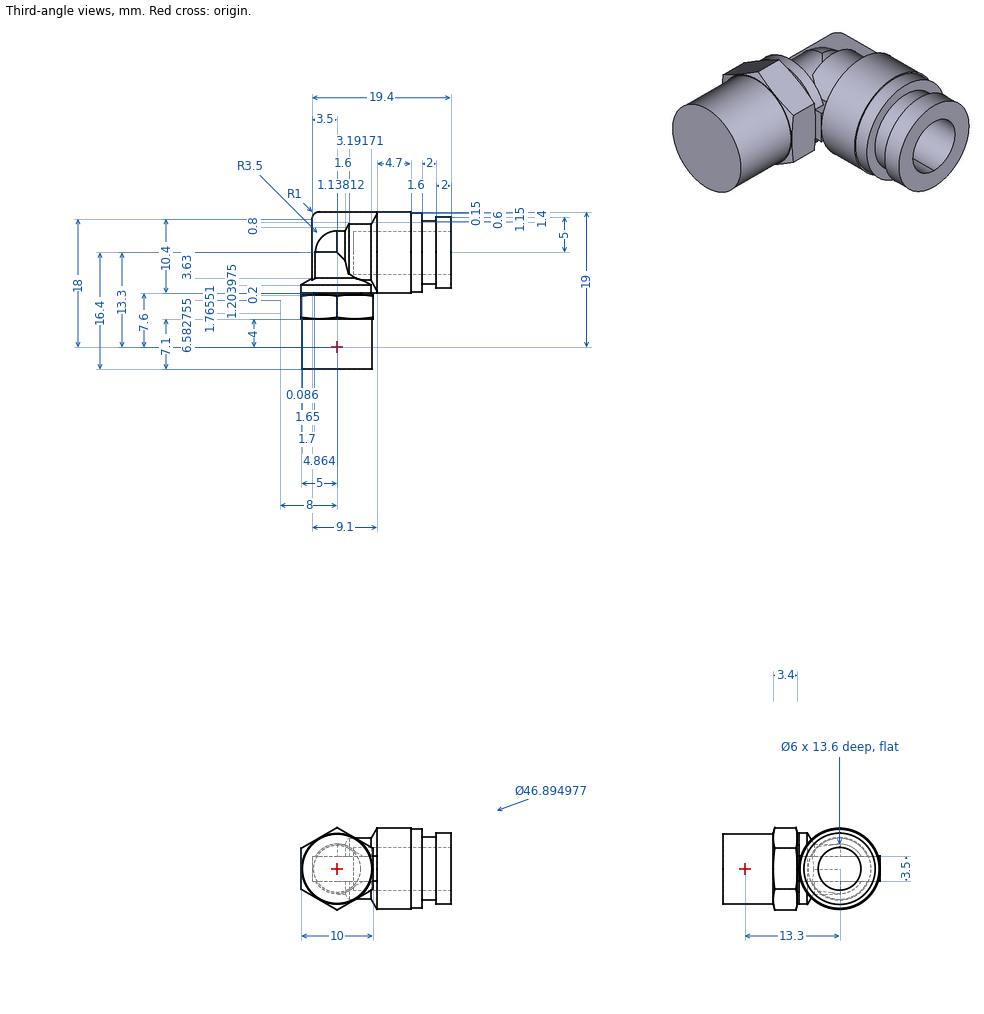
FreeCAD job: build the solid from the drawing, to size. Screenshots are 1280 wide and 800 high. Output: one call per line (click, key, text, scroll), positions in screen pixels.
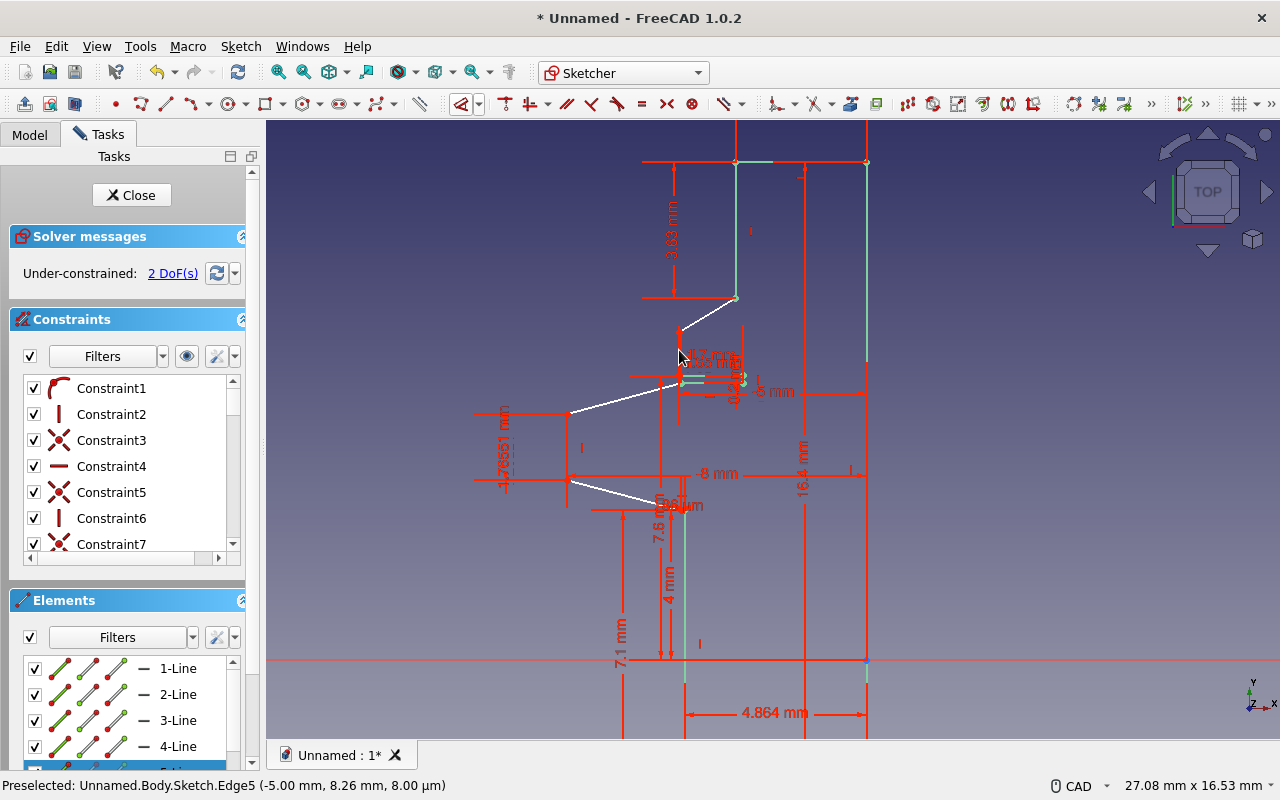
key(i)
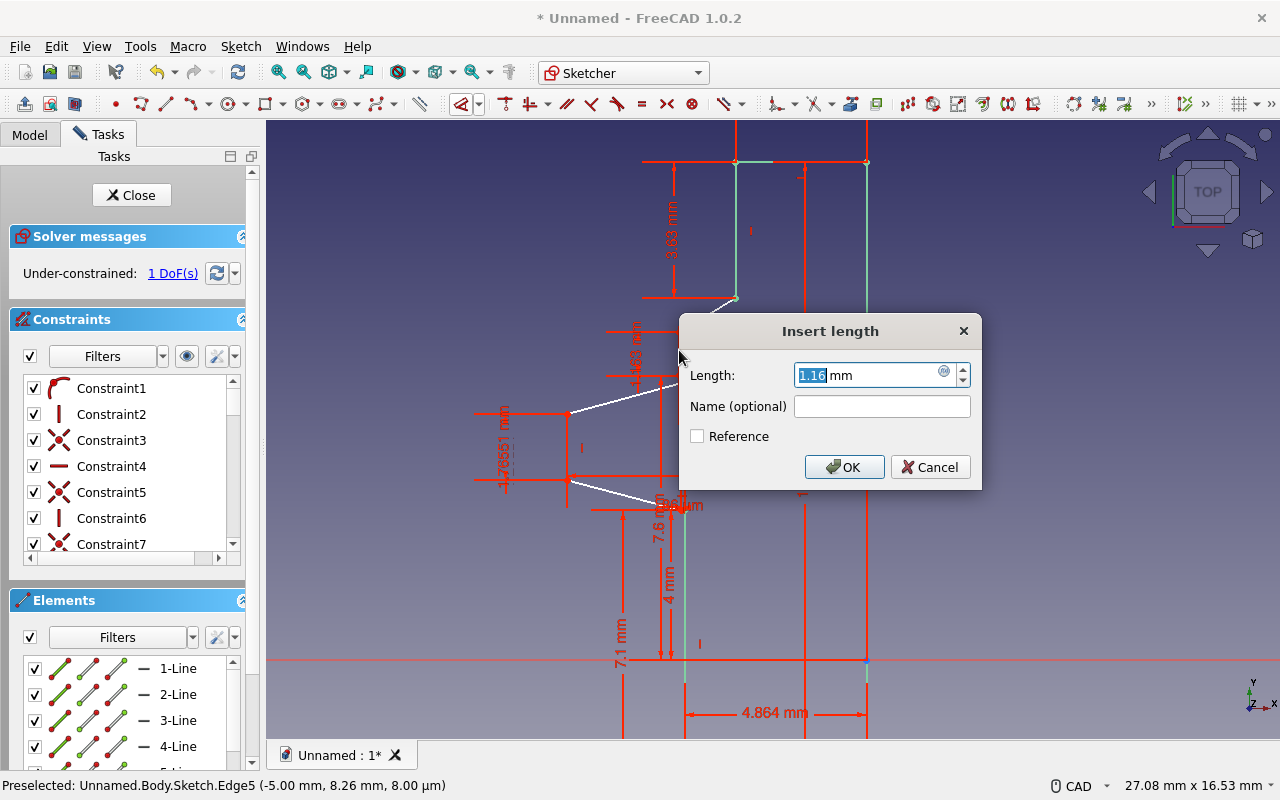
text(1.203975)
key(Return)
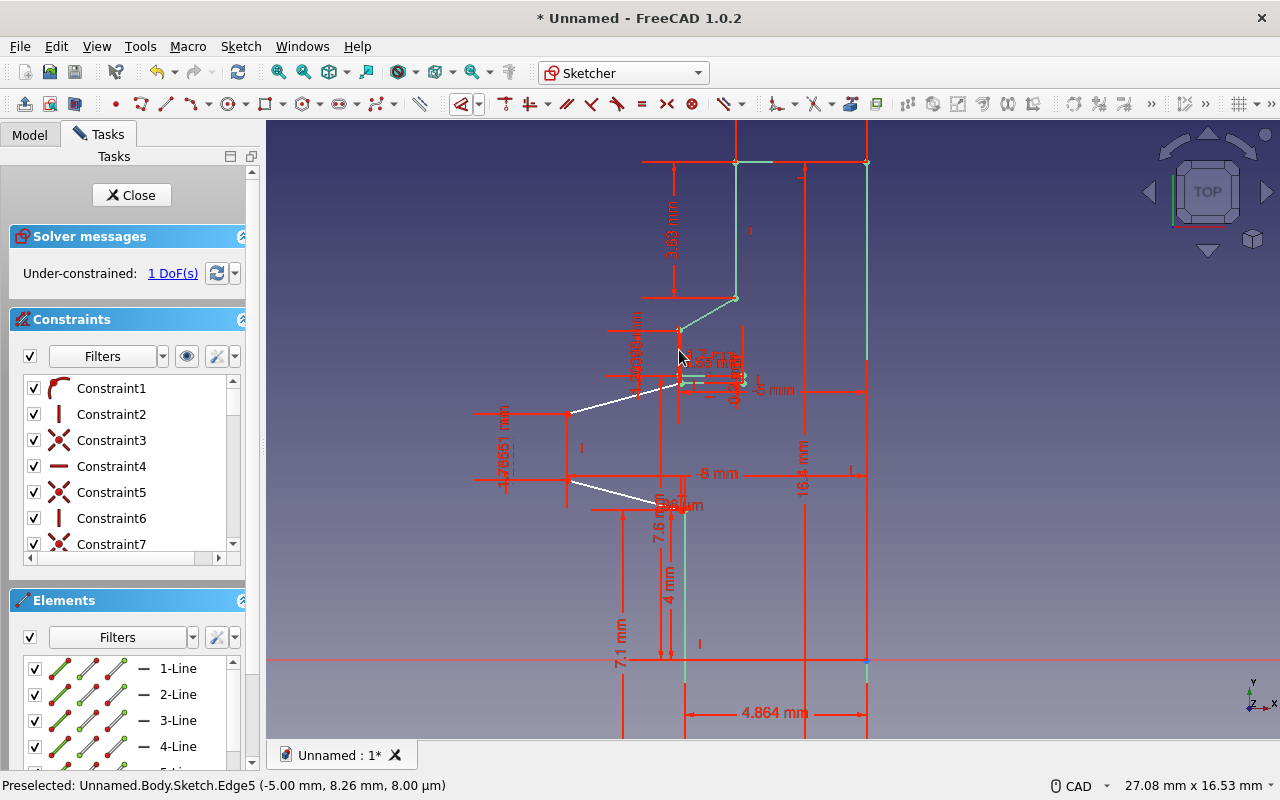
click(567, 414)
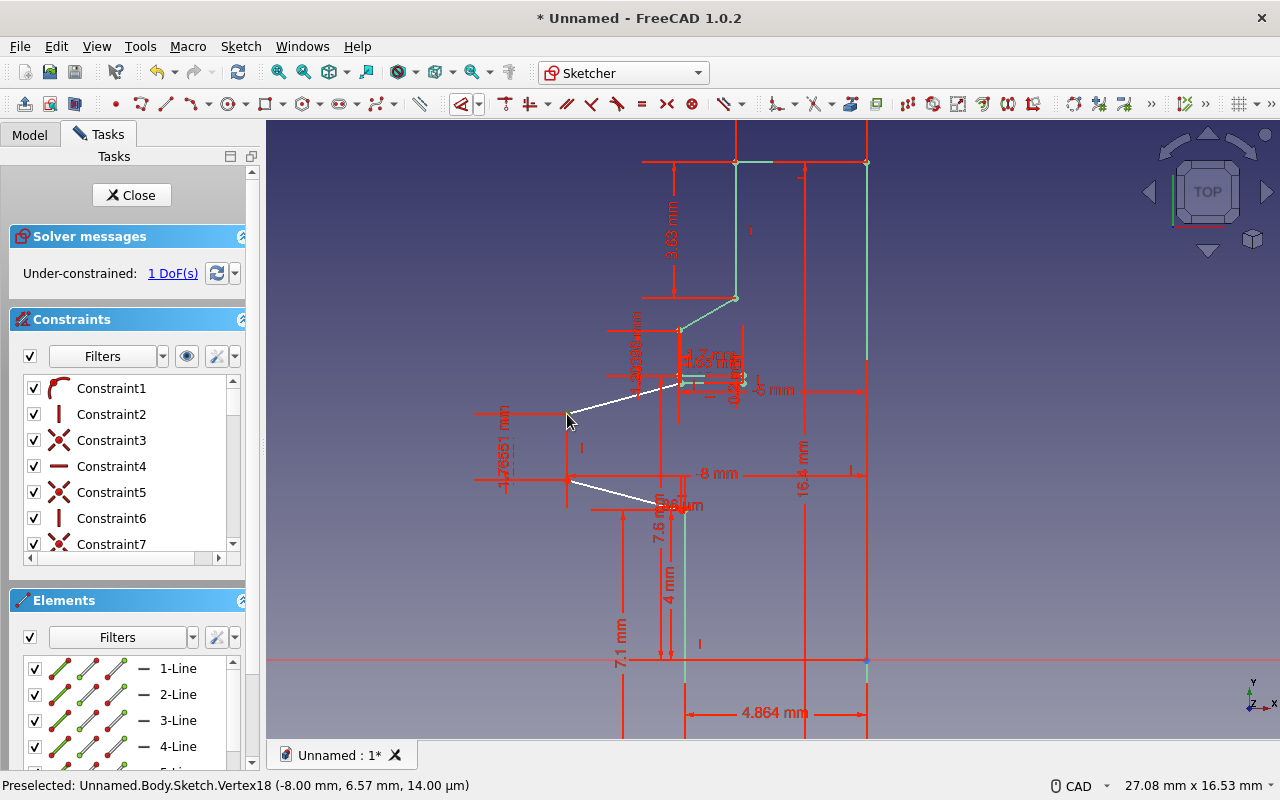
key(i)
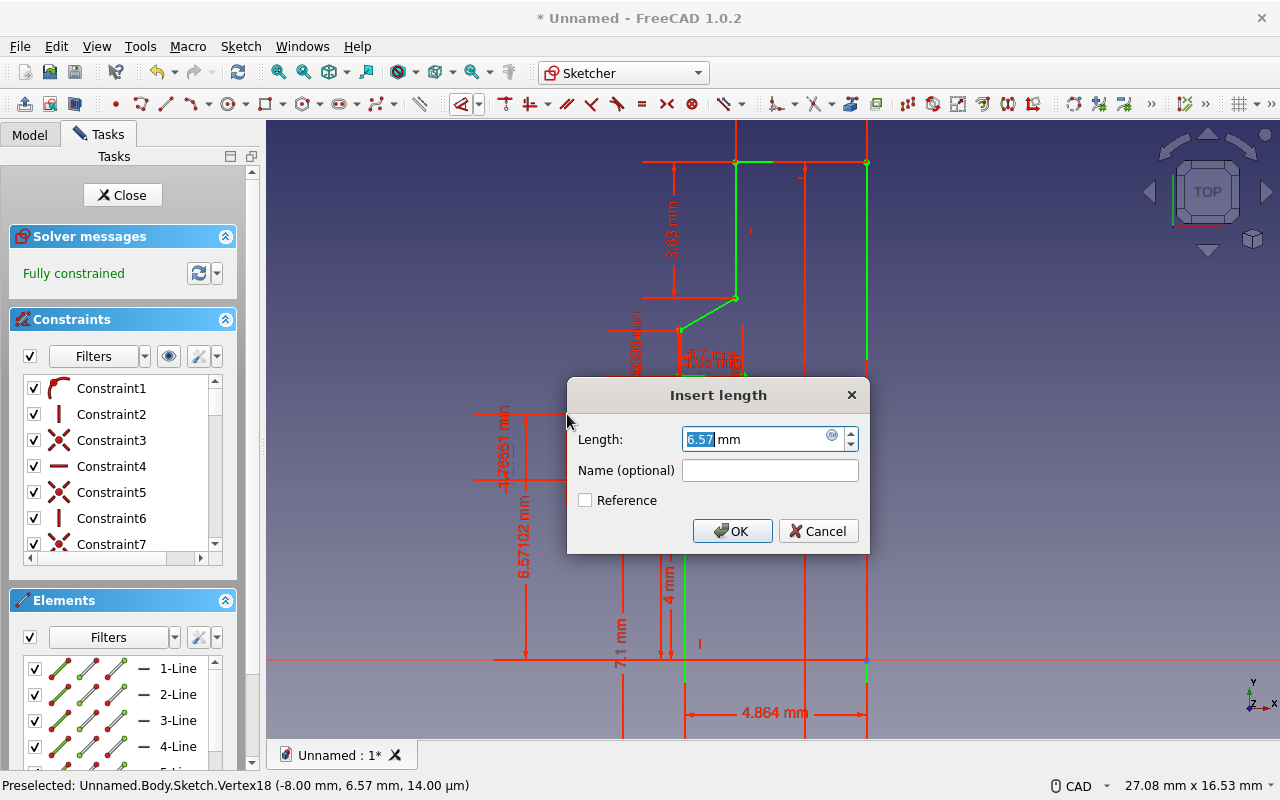
text(6.582755)
key(Return)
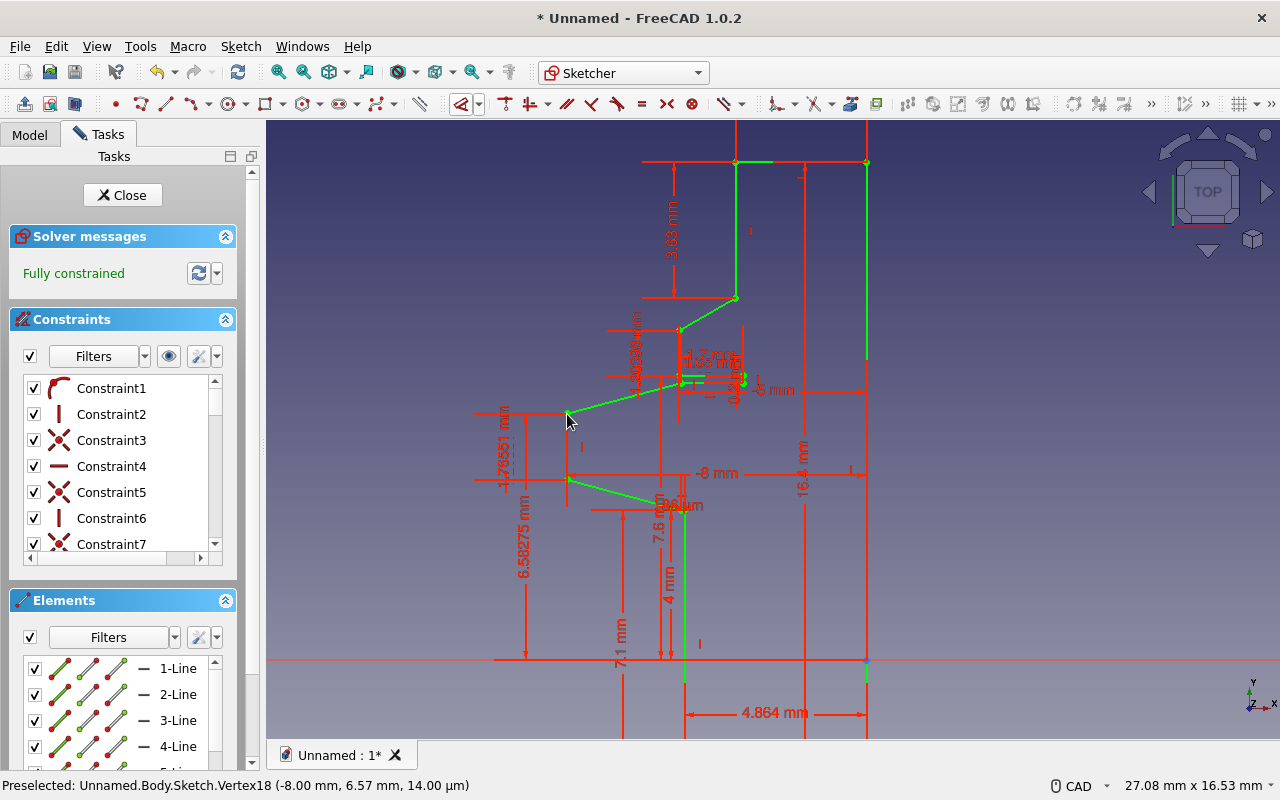
click(123, 195)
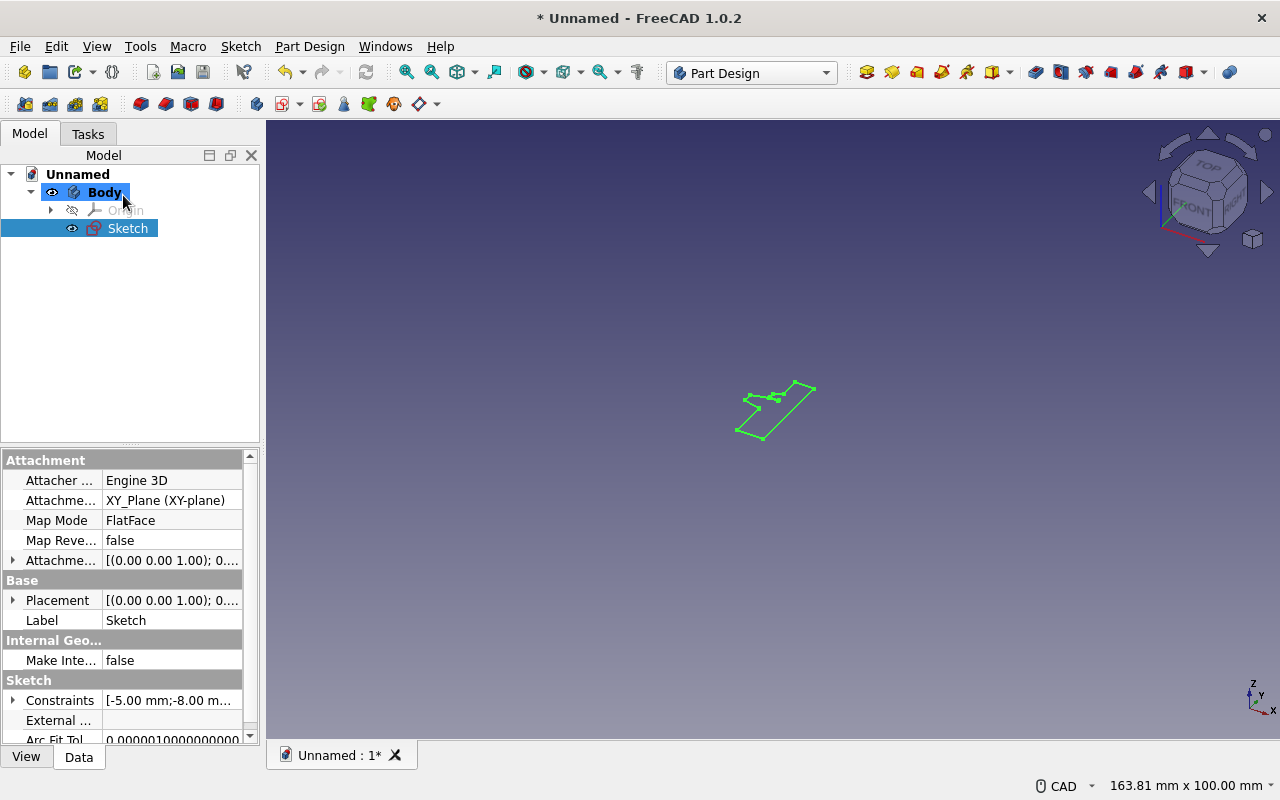
click(892, 72)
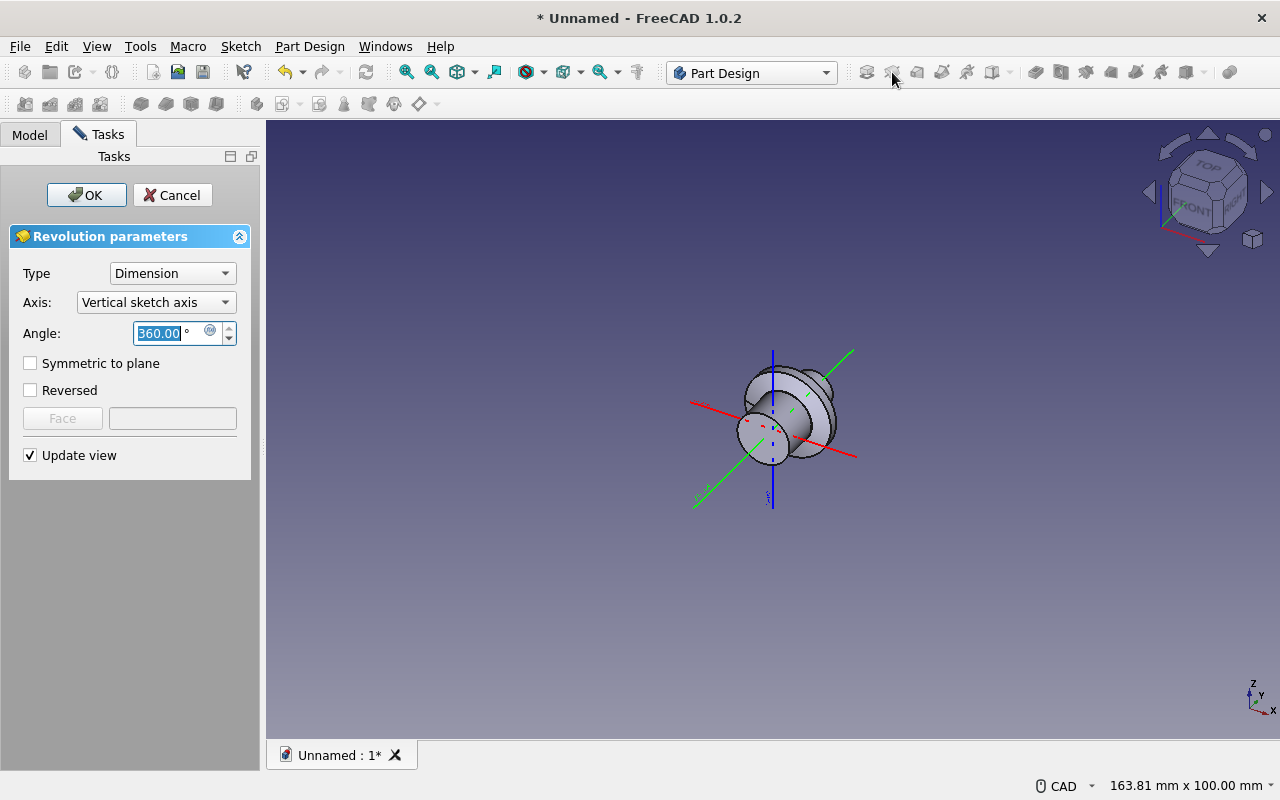
click(87, 195)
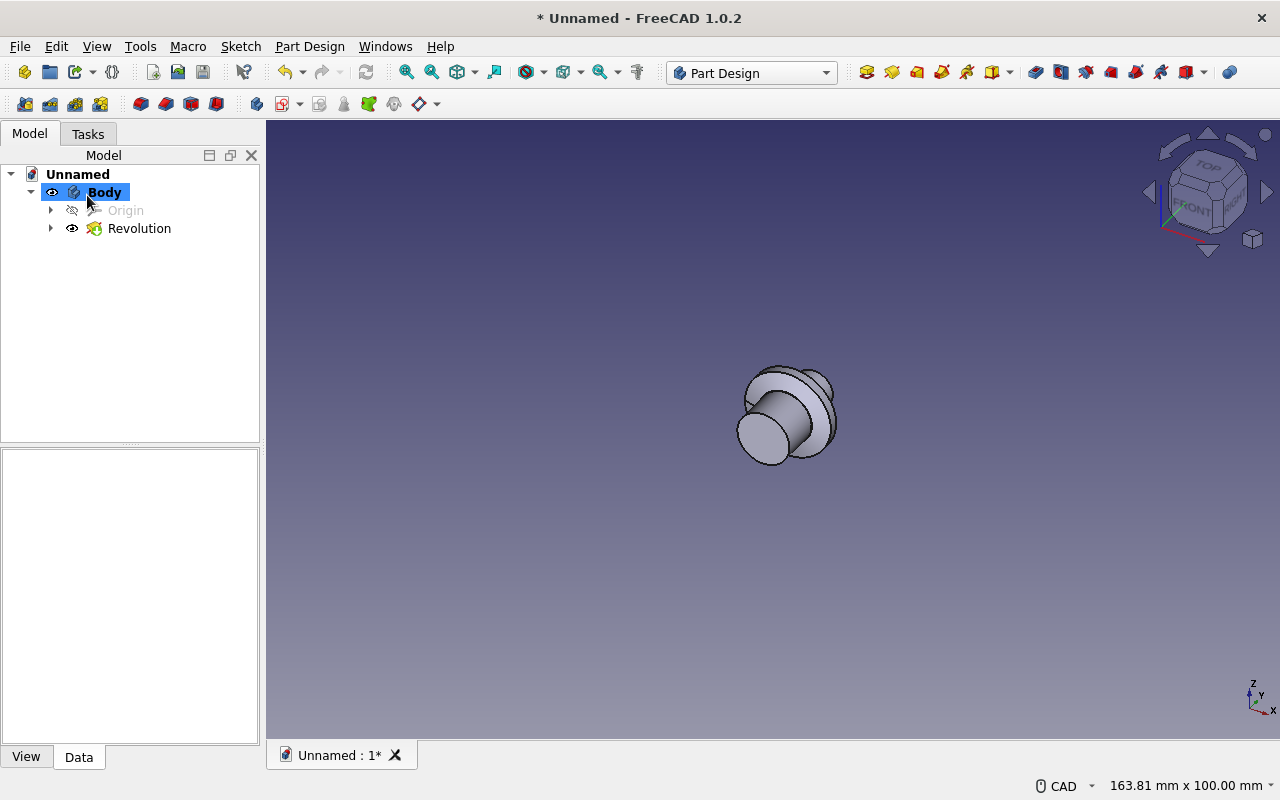
key(v)
key(f)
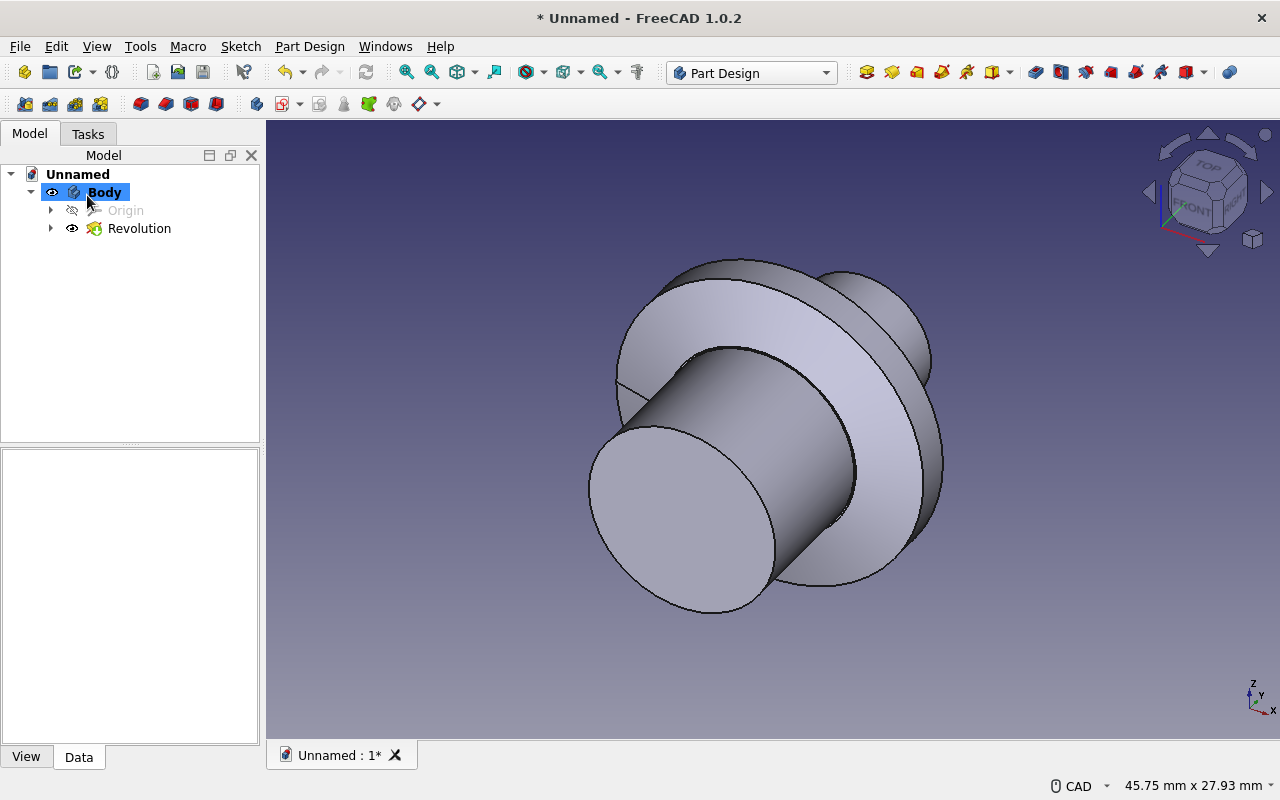
click(282, 104)